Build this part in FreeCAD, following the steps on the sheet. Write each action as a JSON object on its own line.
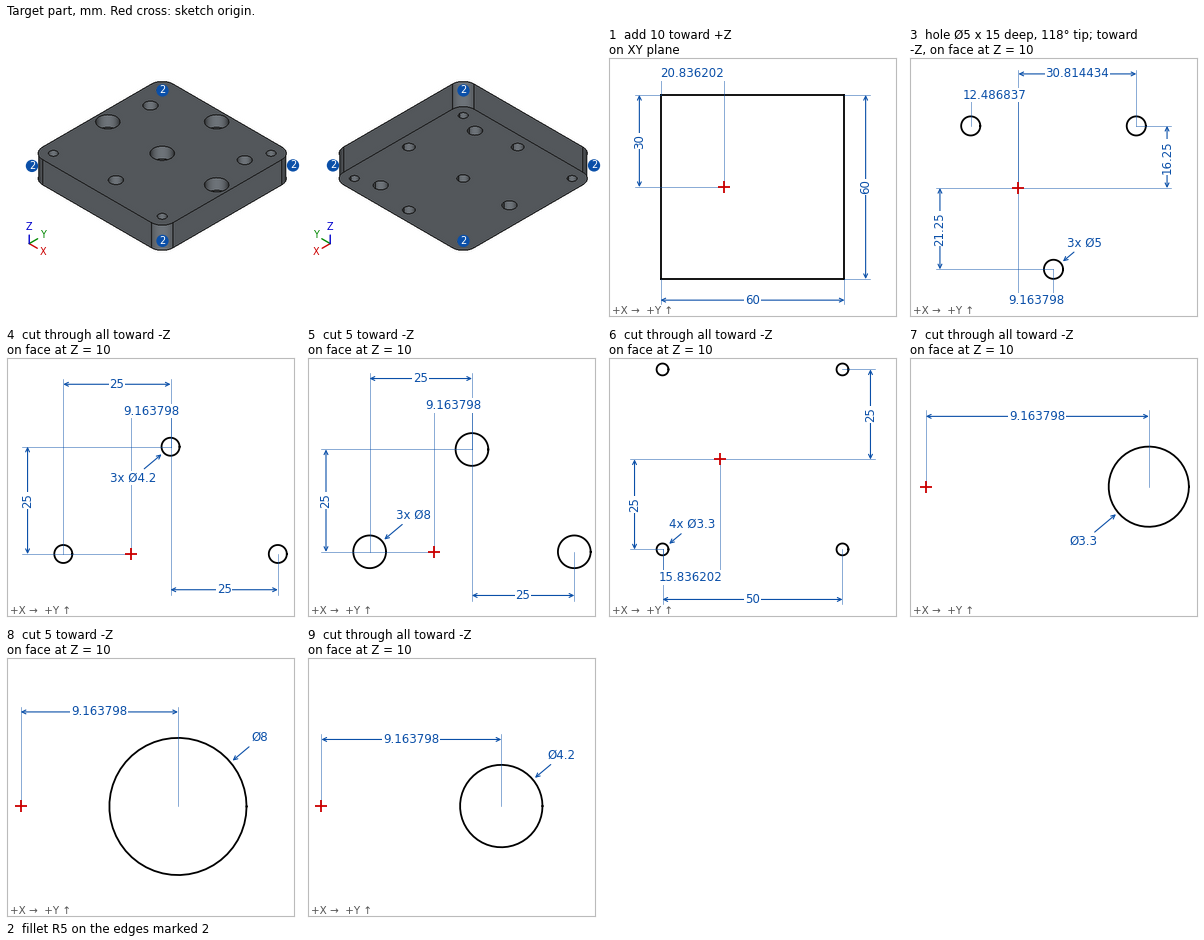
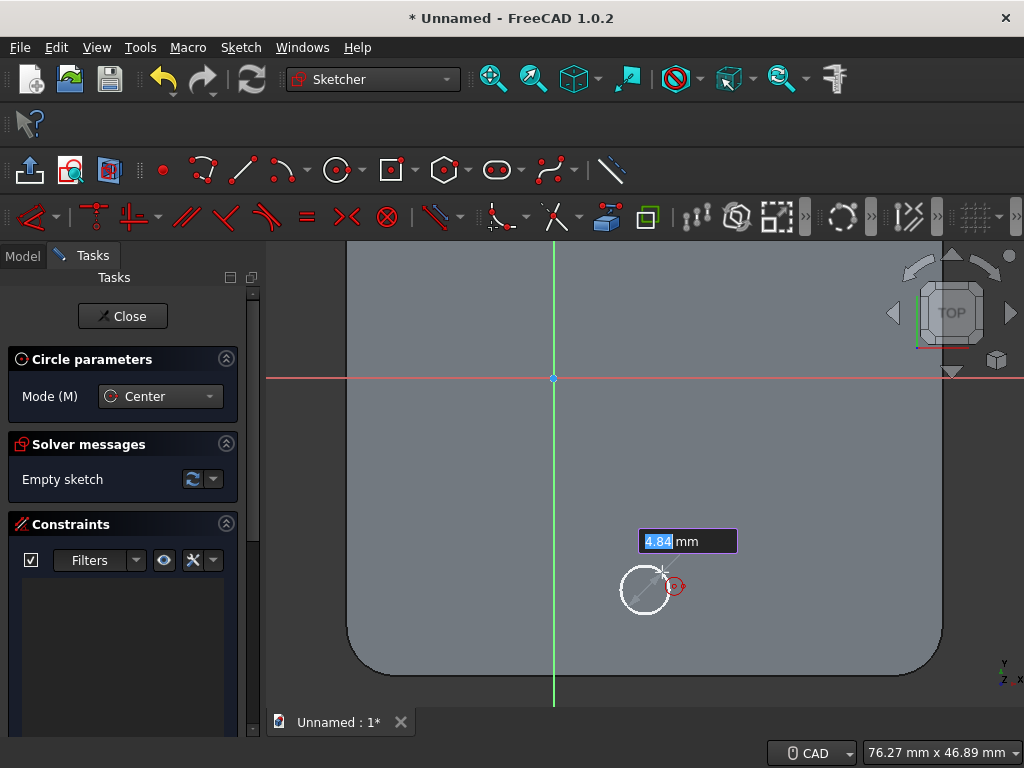
{"action": "type", "text": "5"}
{"action": "key", "text": "Return"}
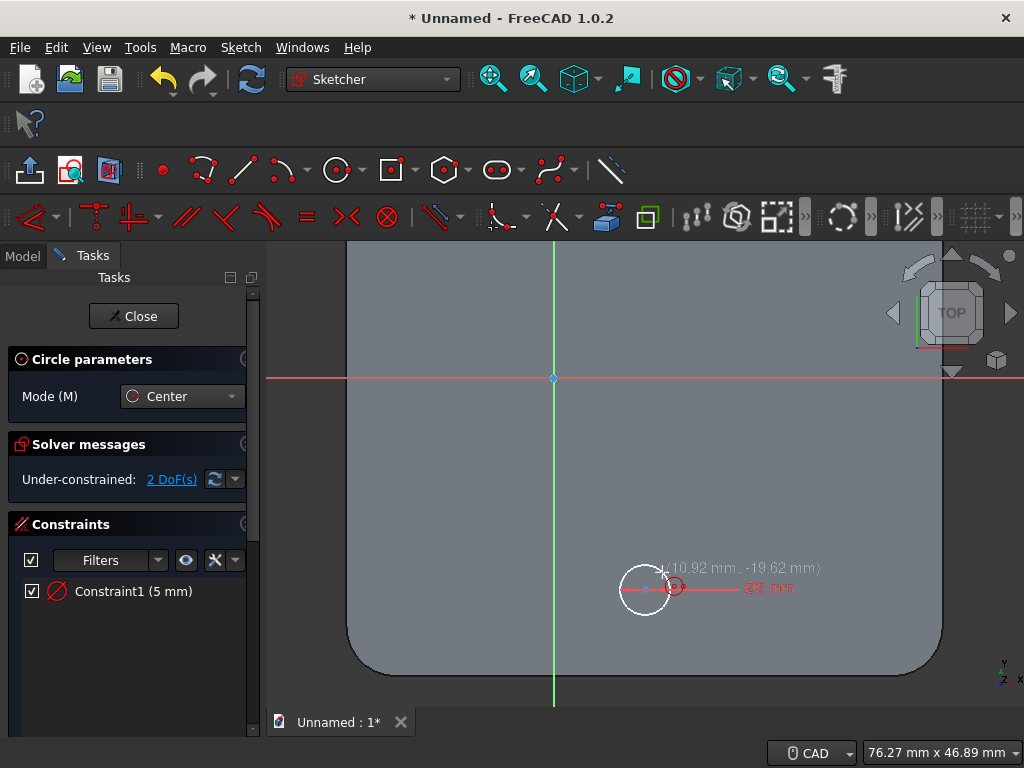
{"action": "scroll", "coordinate": [438, 619], "scroll_direction": "down", "scroll_amount": 2}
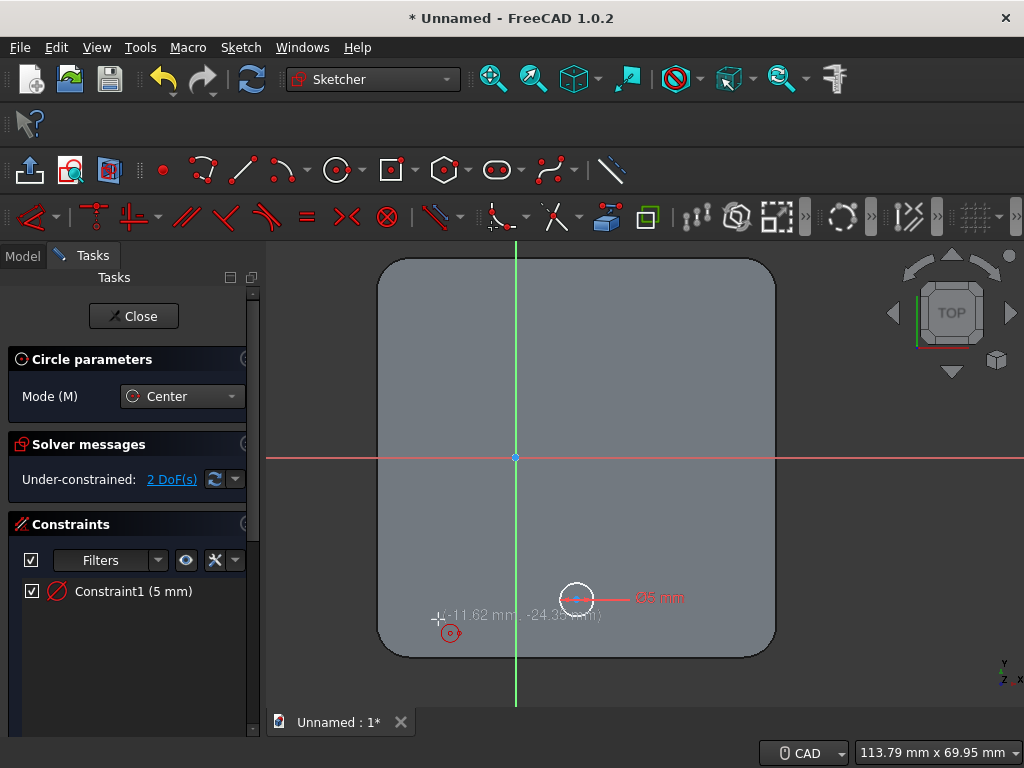
{"action": "scroll", "coordinate": [721, 349], "scroll_direction": "up", "scroll_amount": 2}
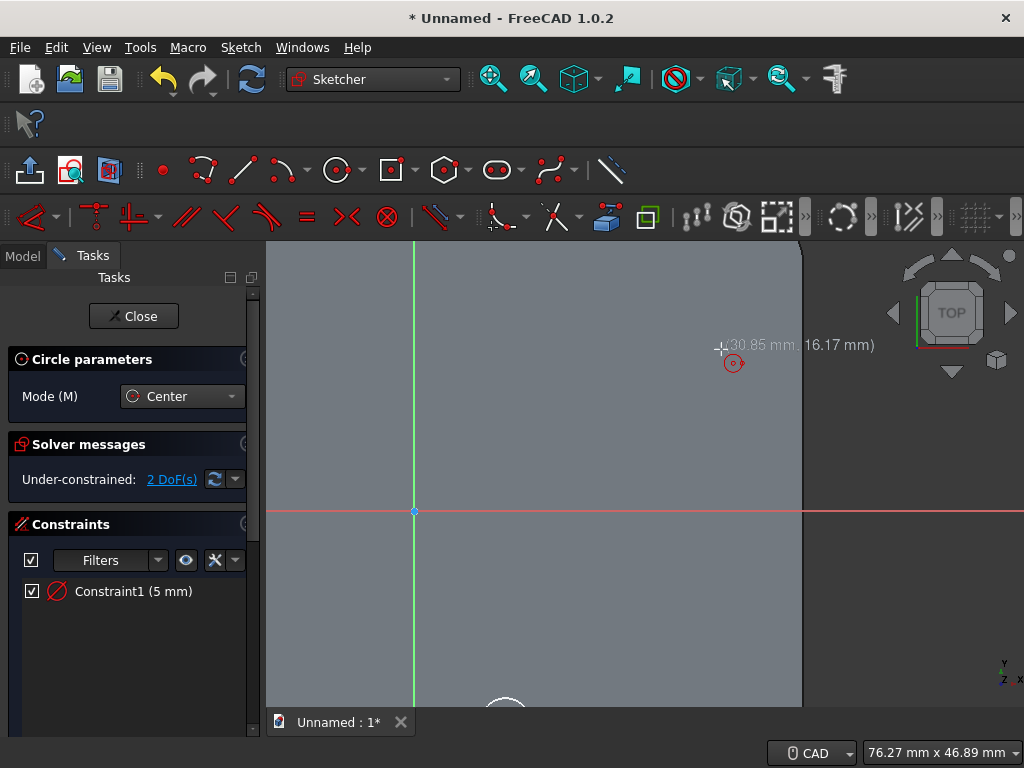
{"action": "left_click", "coordinate": [720, 350]}
{"action": "mouse_move", "coordinate": [738, 332]}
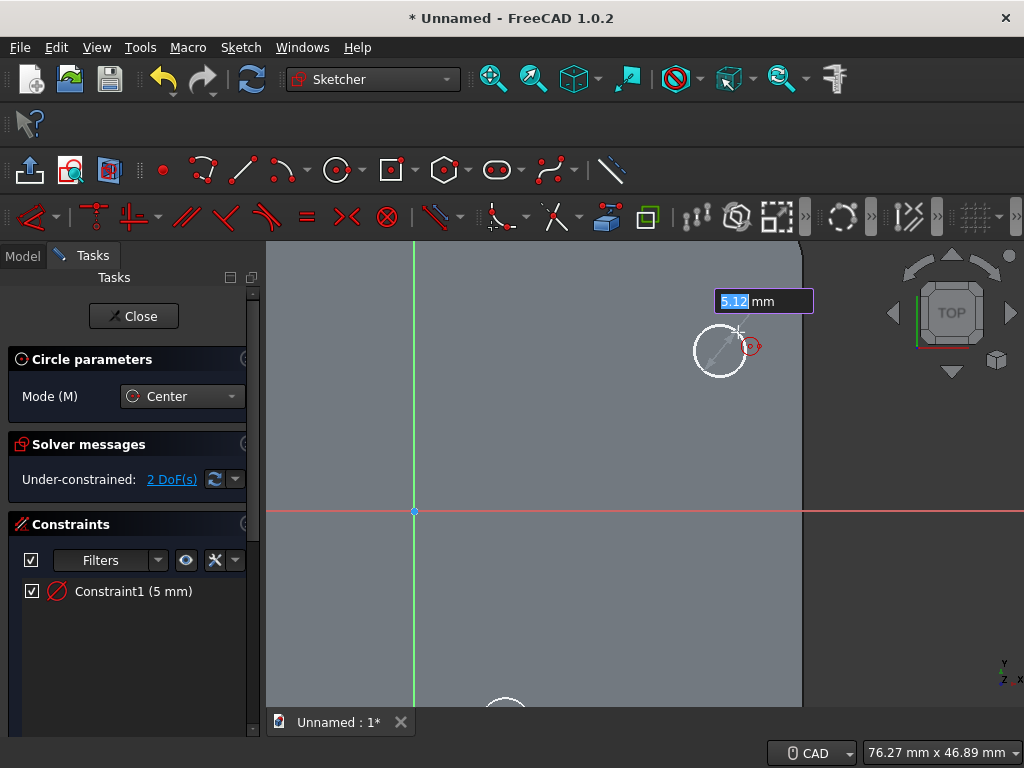
{"action": "type", "text": "5"}
{"action": "key", "text": "Return"}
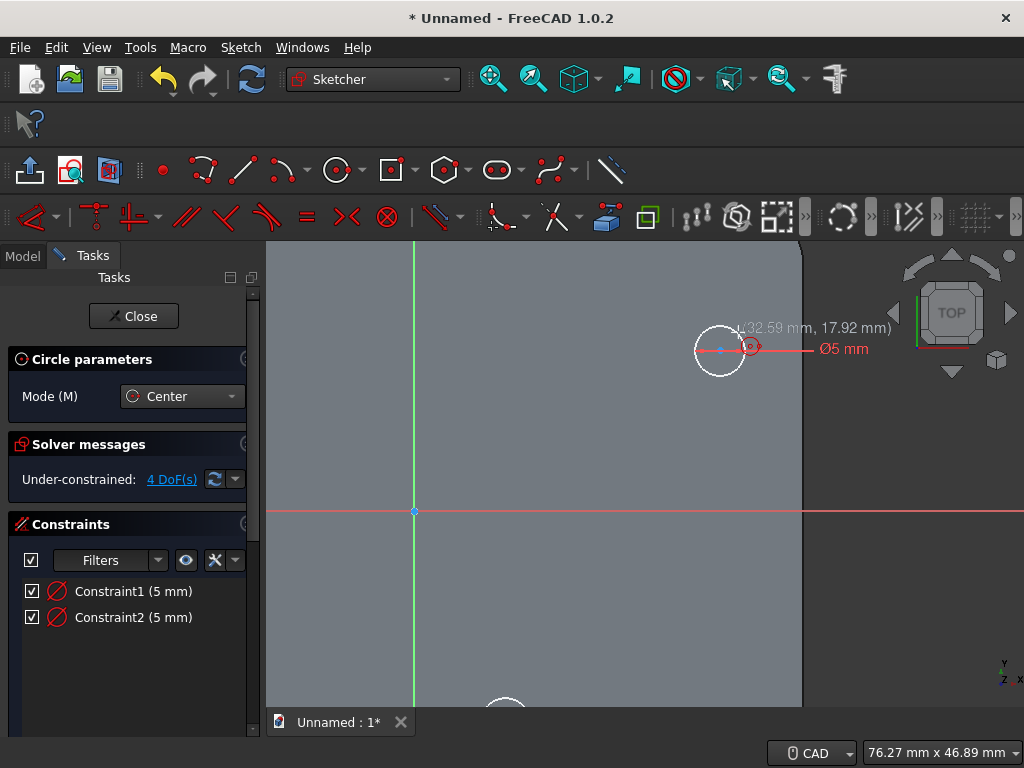
{"action": "scroll", "coordinate": [721, 348], "scroll_direction": "down", "scroll_amount": 2}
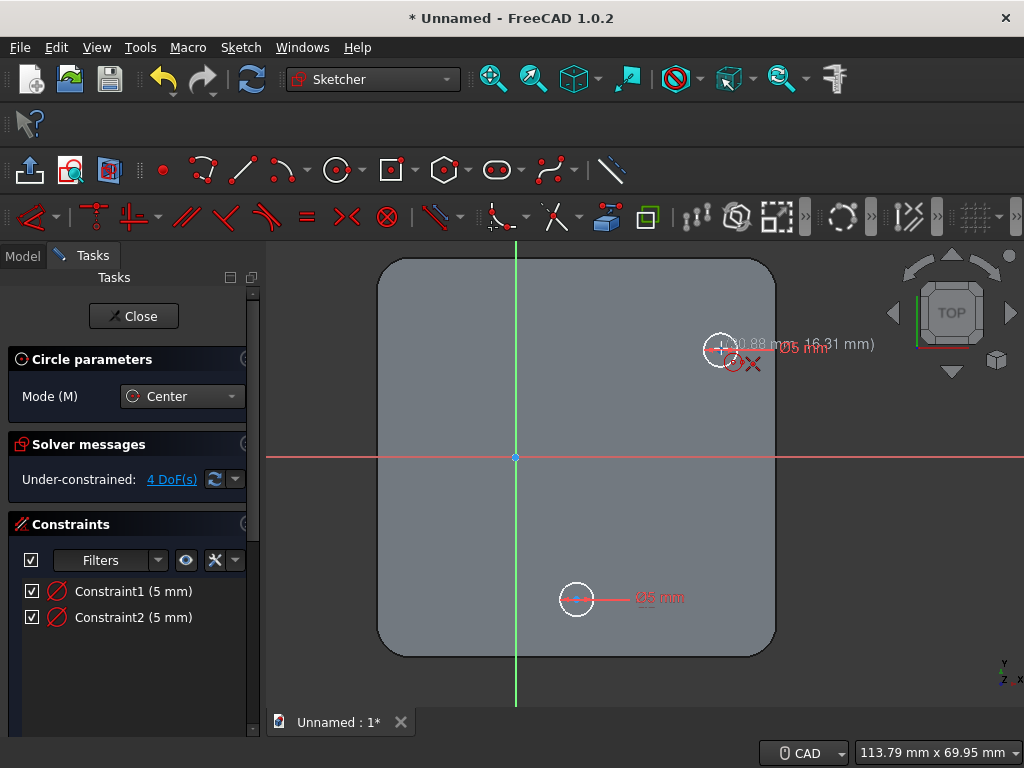
{"action": "scroll", "coordinate": [432, 349], "scroll_direction": "up", "scroll_amount": 2}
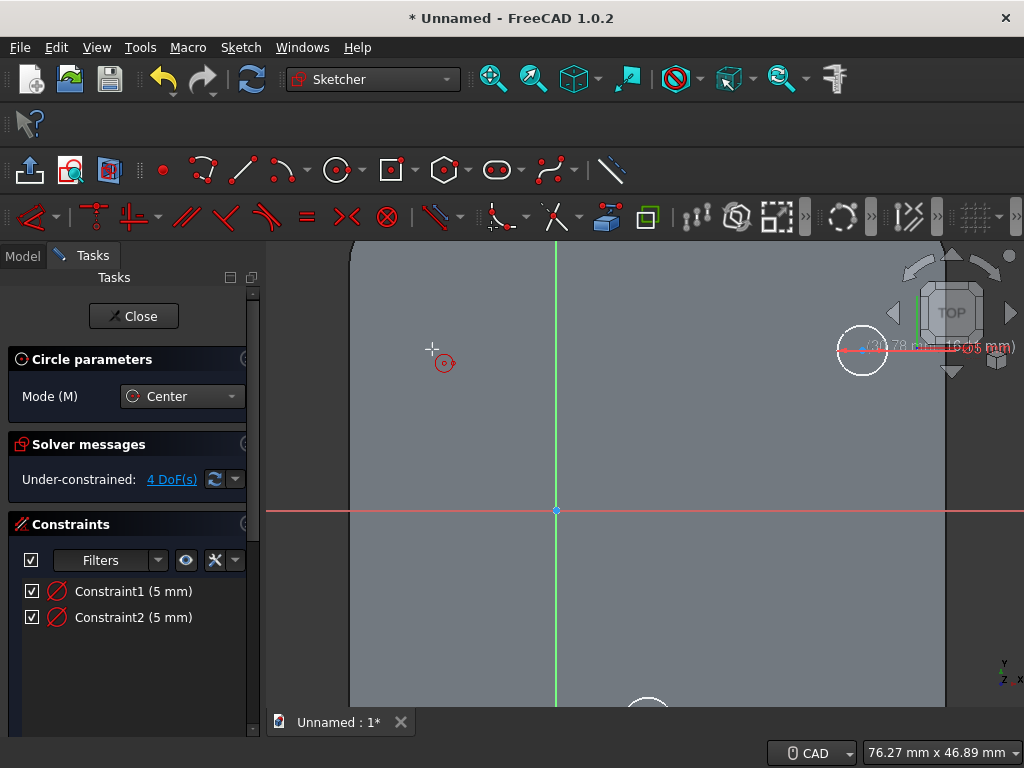
{"action": "left_click", "coordinate": [432, 349]}
{"action": "mouse_move", "coordinate": [450, 332]}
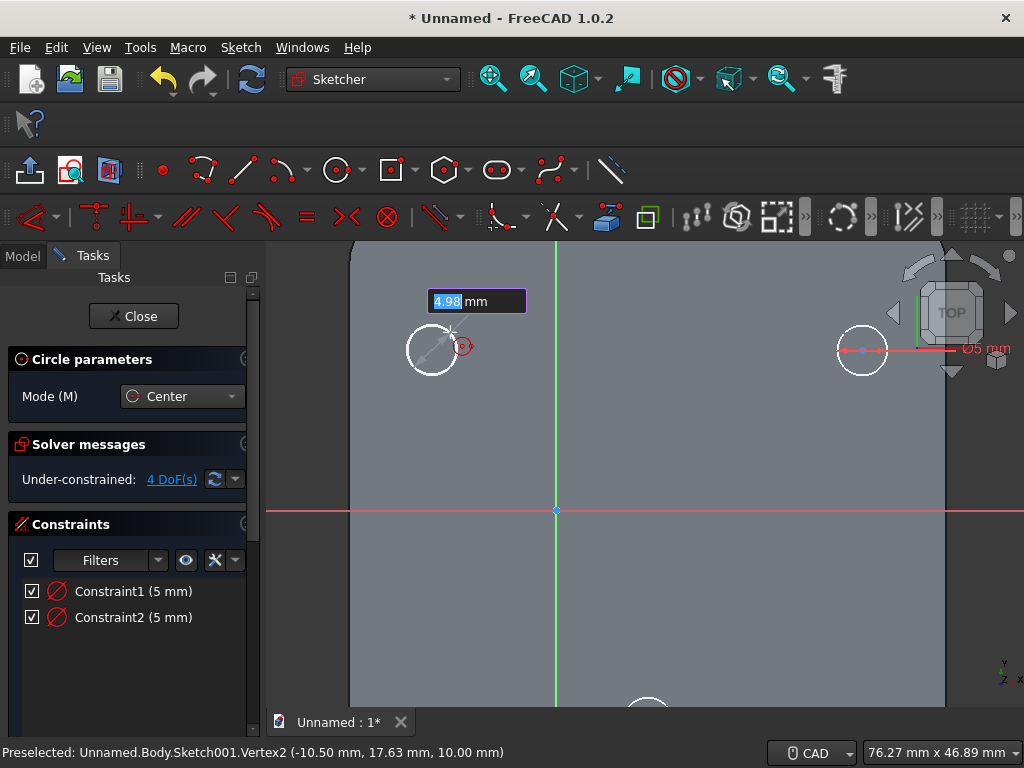
{"action": "type", "text": "5"}
{"action": "key", "text": "Return"}
{"action": "key", "text": "Escape"}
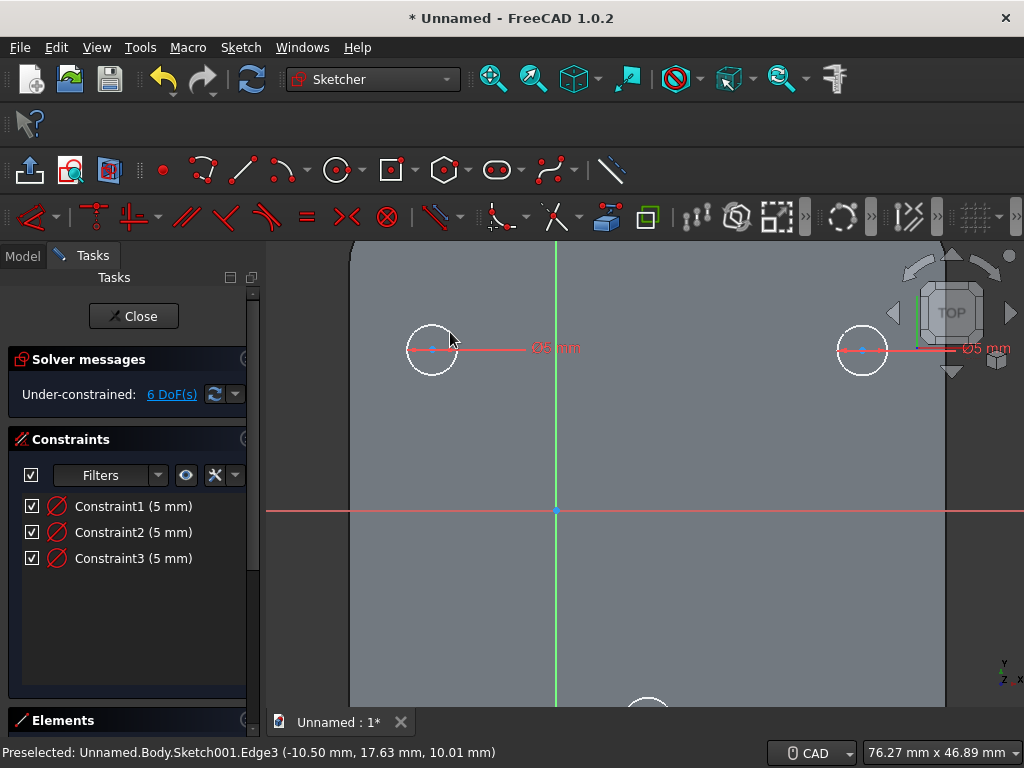
{"action": "scroll", "coordinate": [432, 349], "scroll_direction": "down", "scroll_amount": 2}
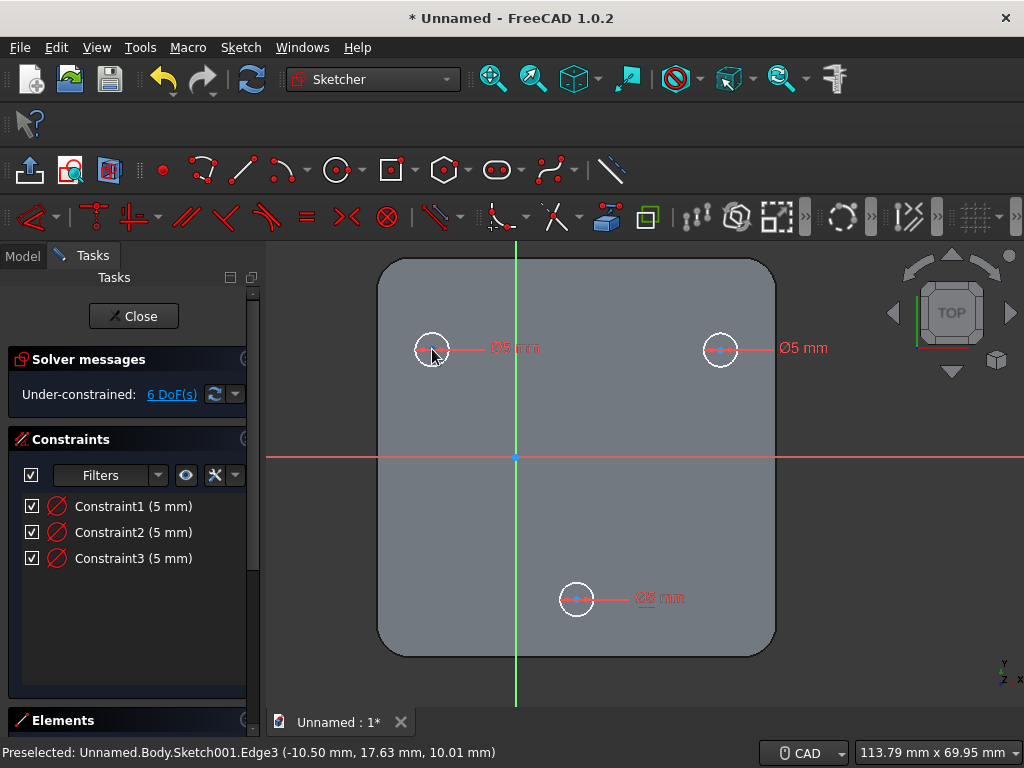
{"action": "left_click", "coordinate": [721, 350]}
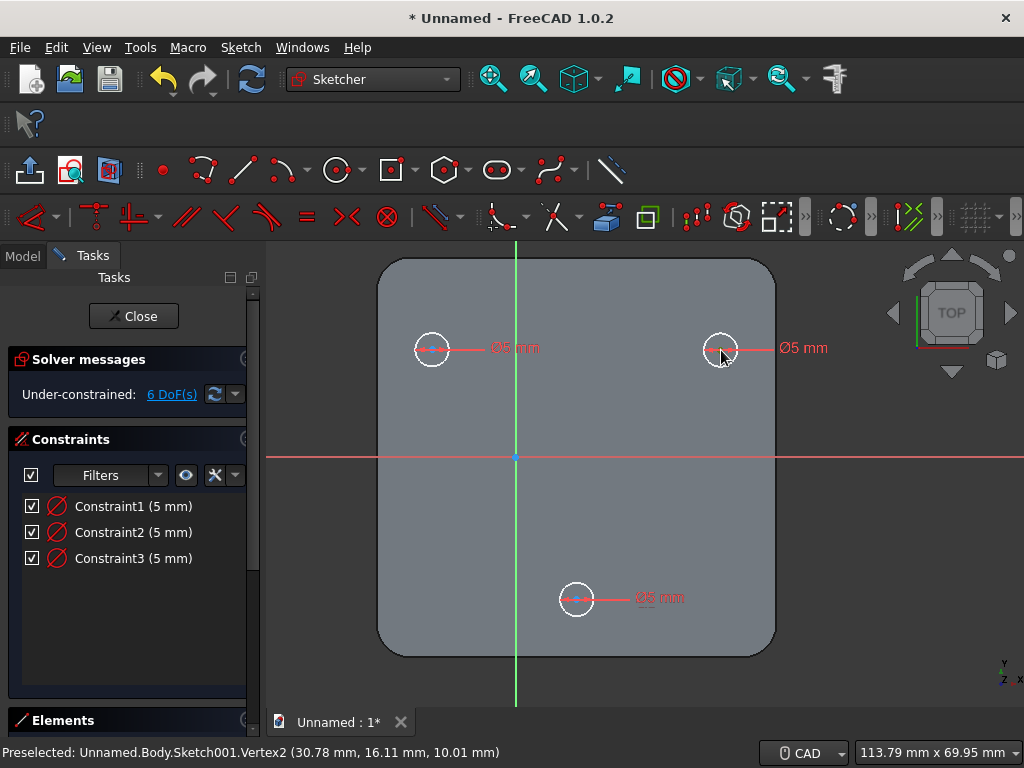
{"action": "left_click", "coordinate": [432, 350]}